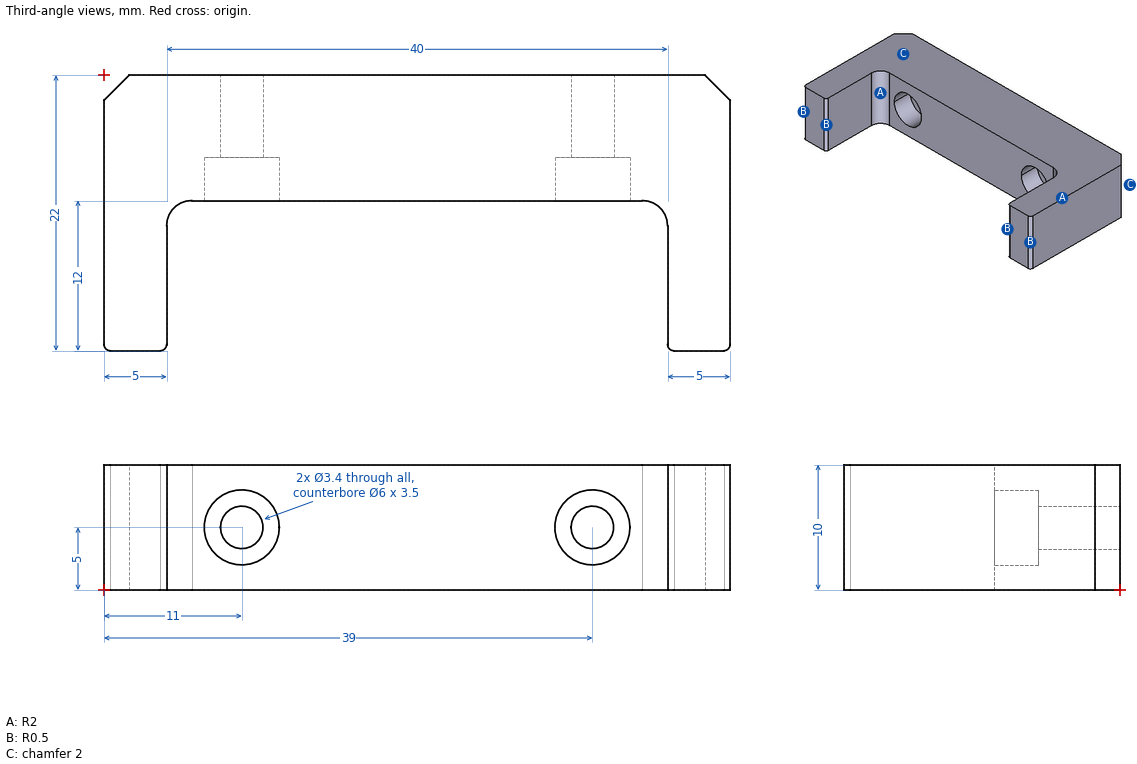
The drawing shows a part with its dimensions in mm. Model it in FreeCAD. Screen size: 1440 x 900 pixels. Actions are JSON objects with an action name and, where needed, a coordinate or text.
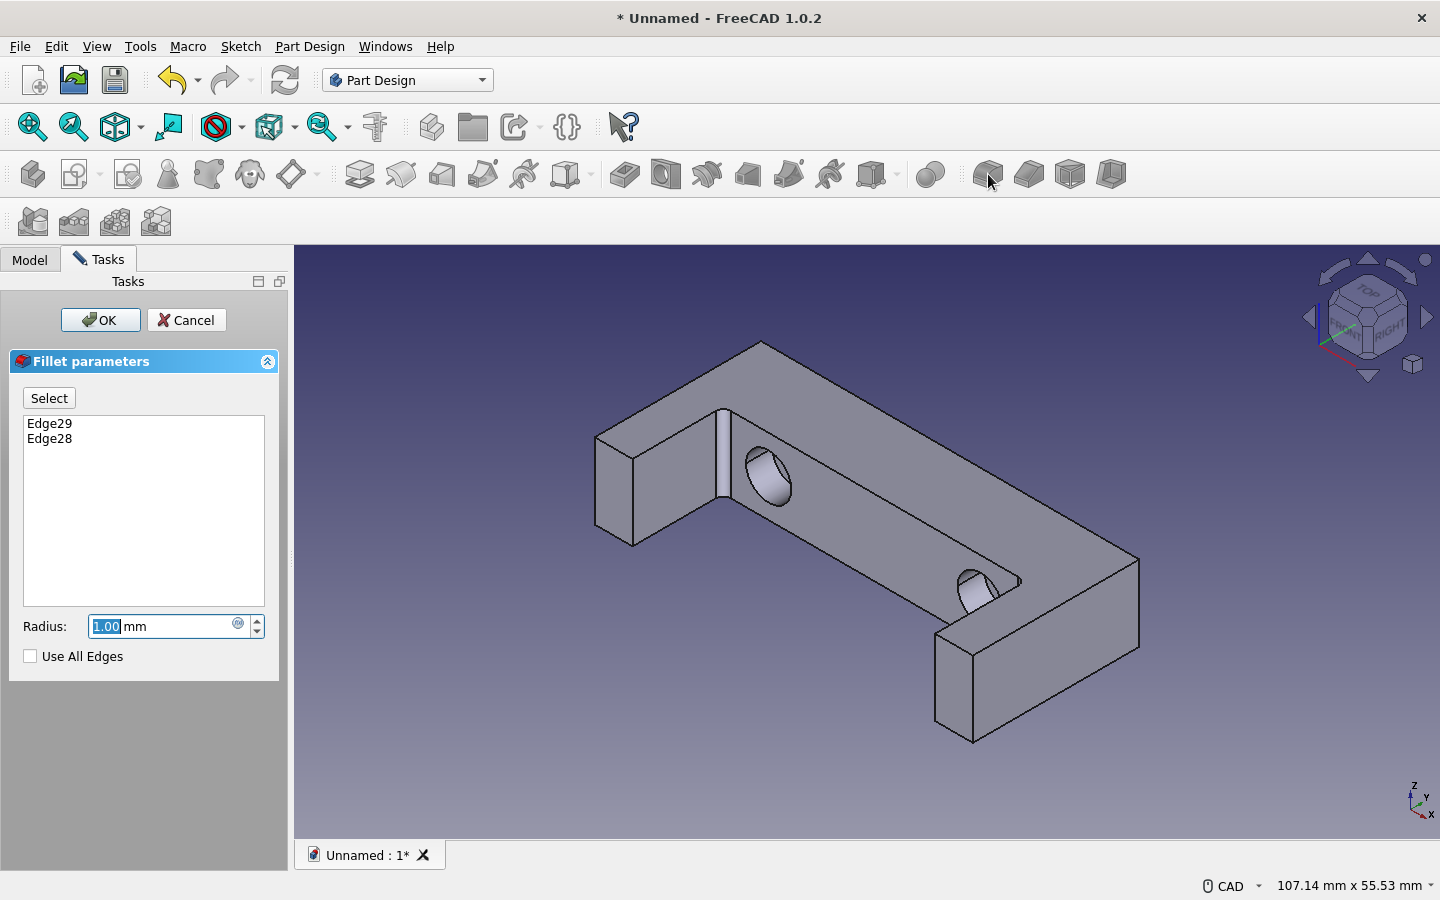
{"action": "type", "text": "2"}
{"action": "key", "text": "Tab"}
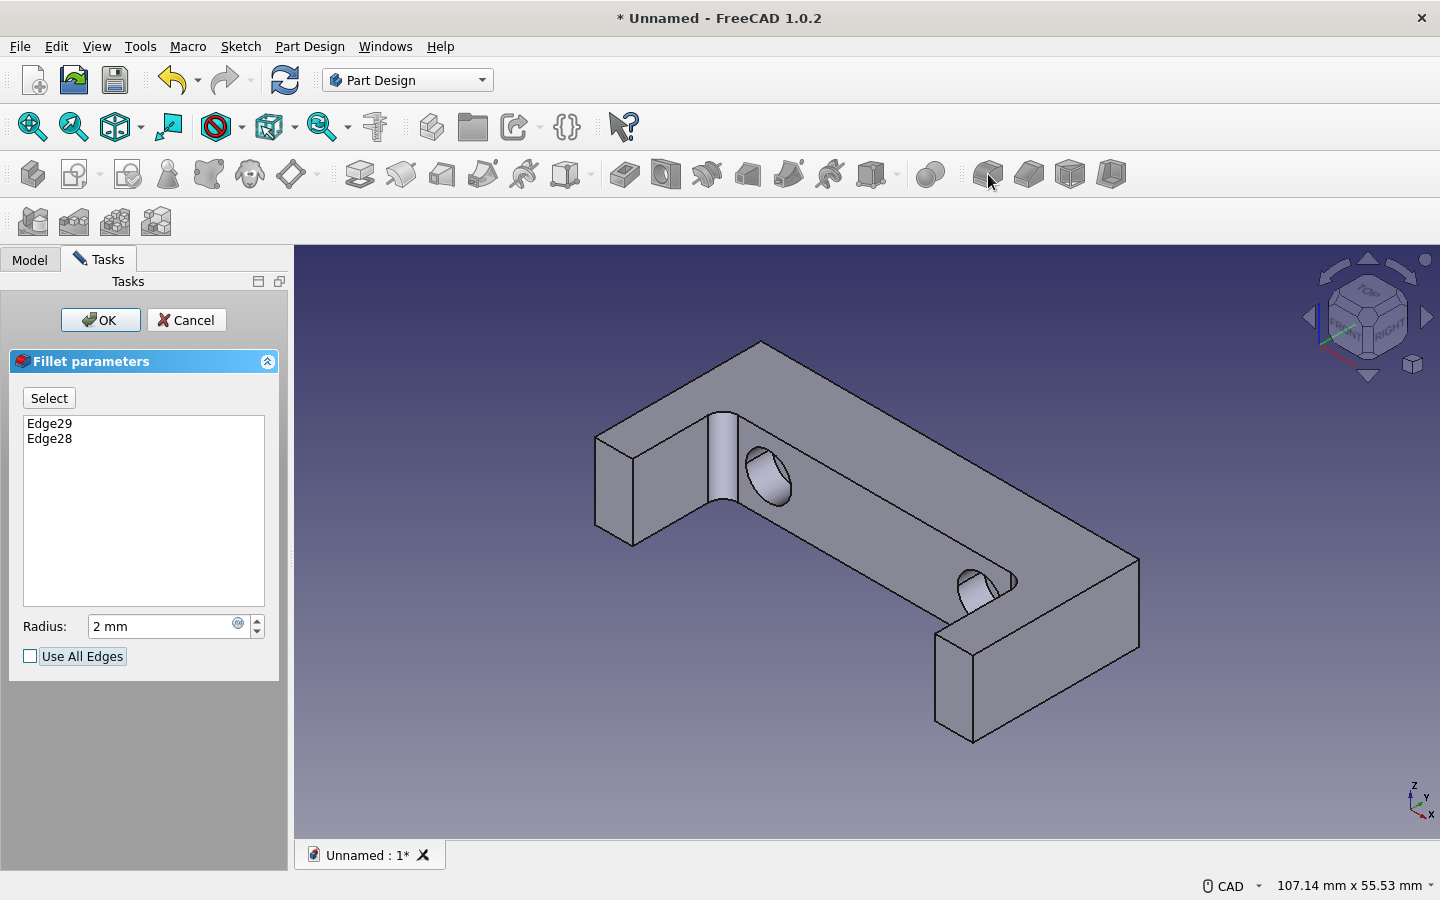
{"action": "left_click", "coordinate": [101, 320]}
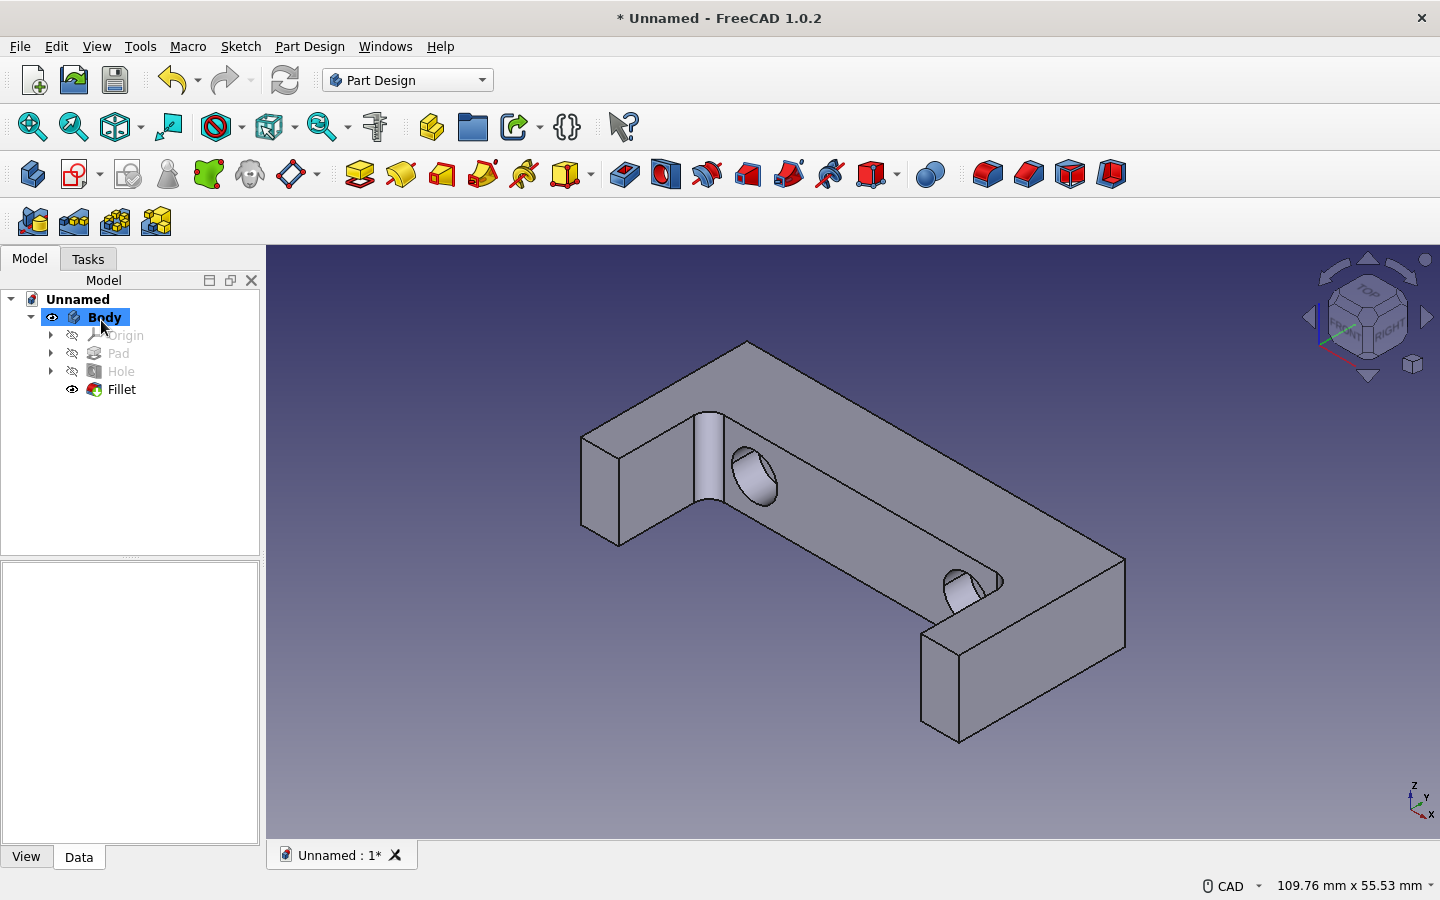
{"action": "left_click", "coordinate": [959, 698]}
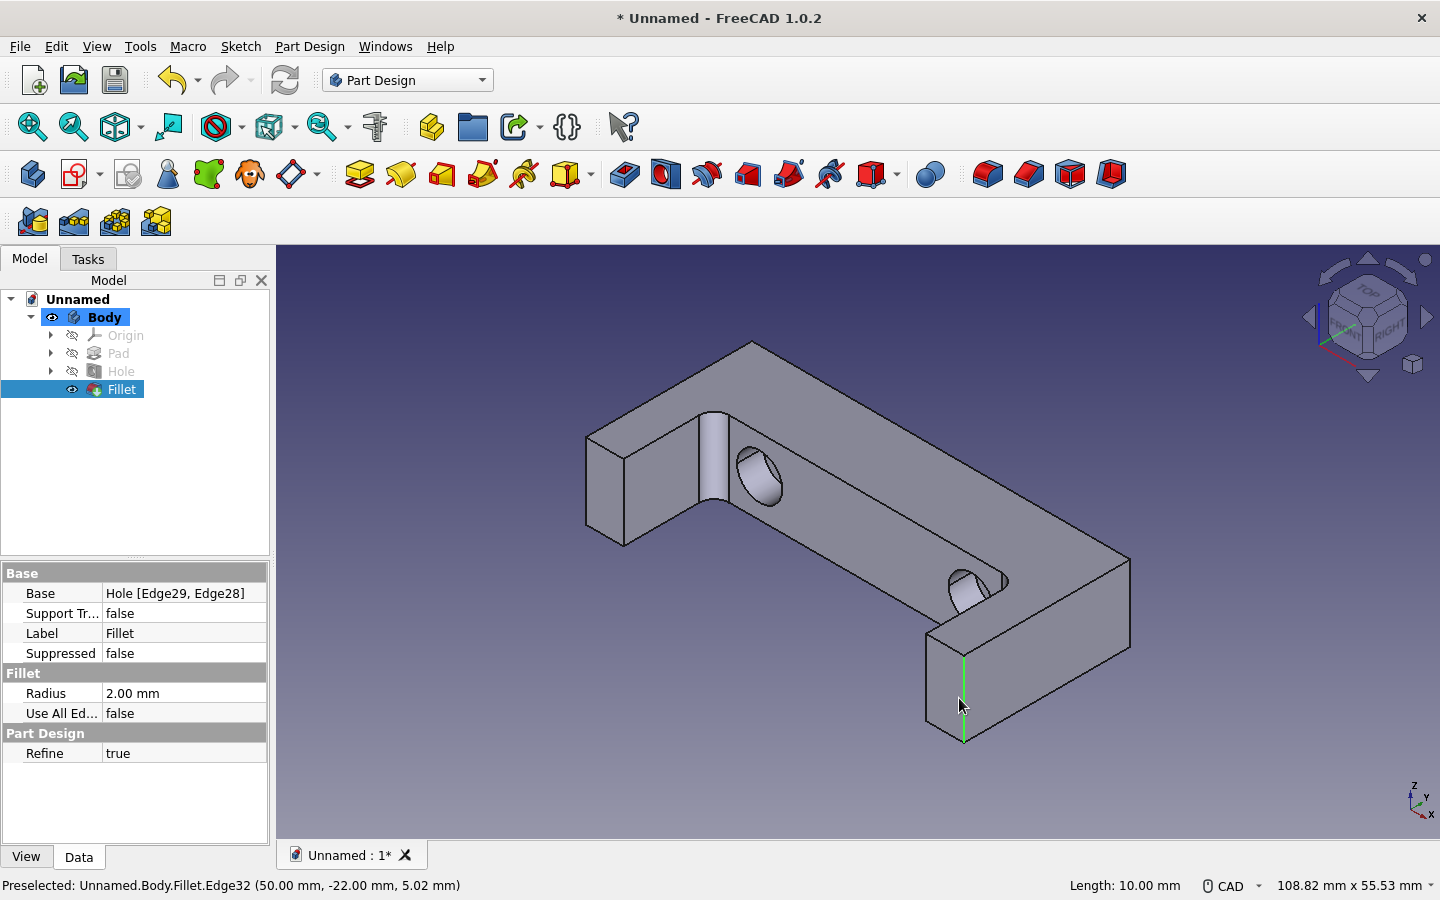
{"action": "left_click", "coordinate": [624, 502], "text": "ctrl"}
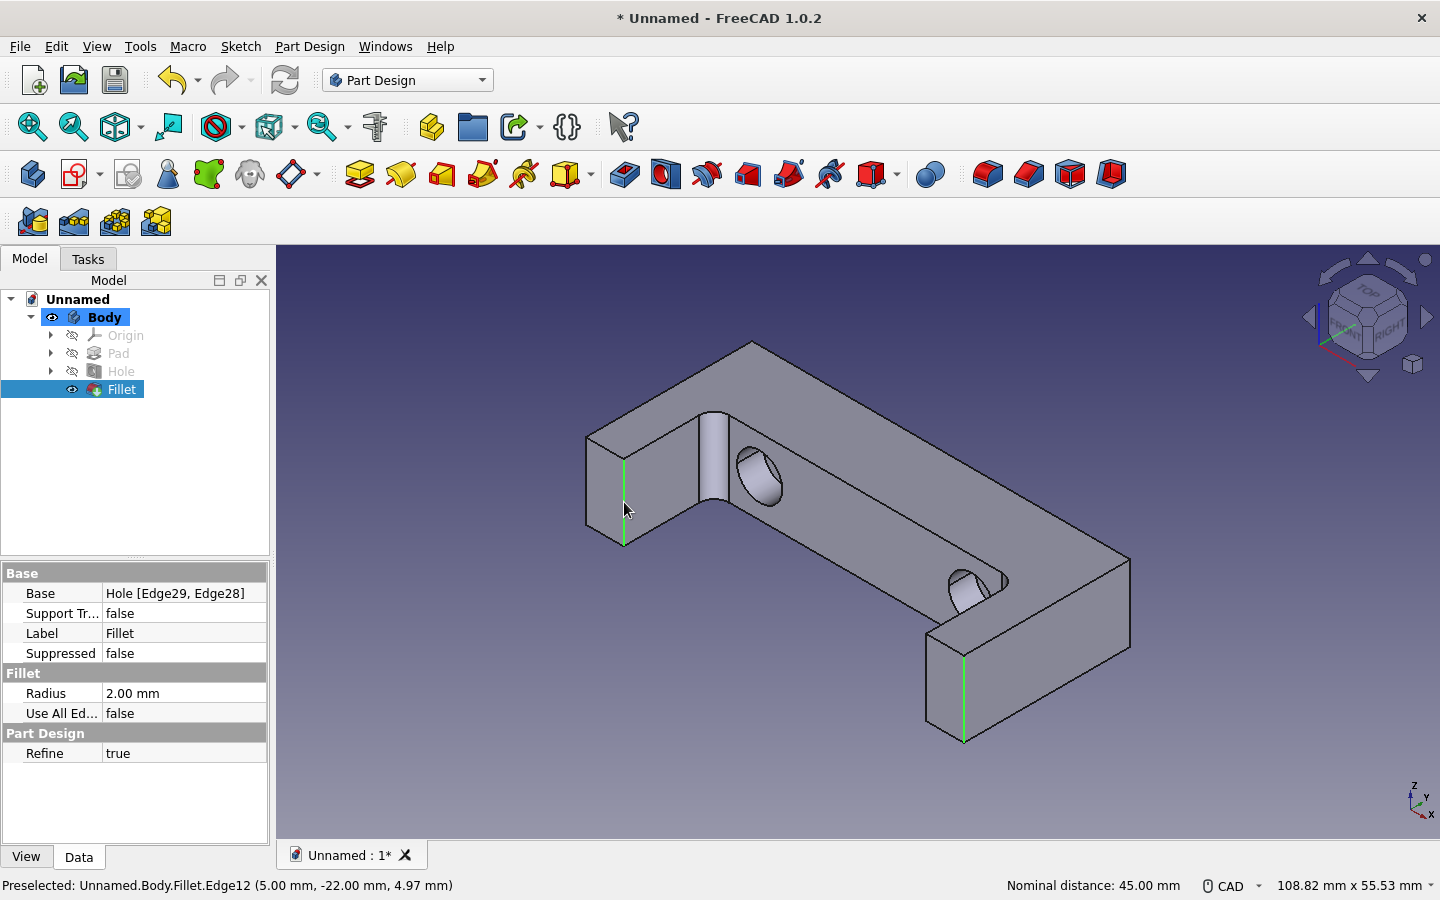
{"action": "key", "text": "2"}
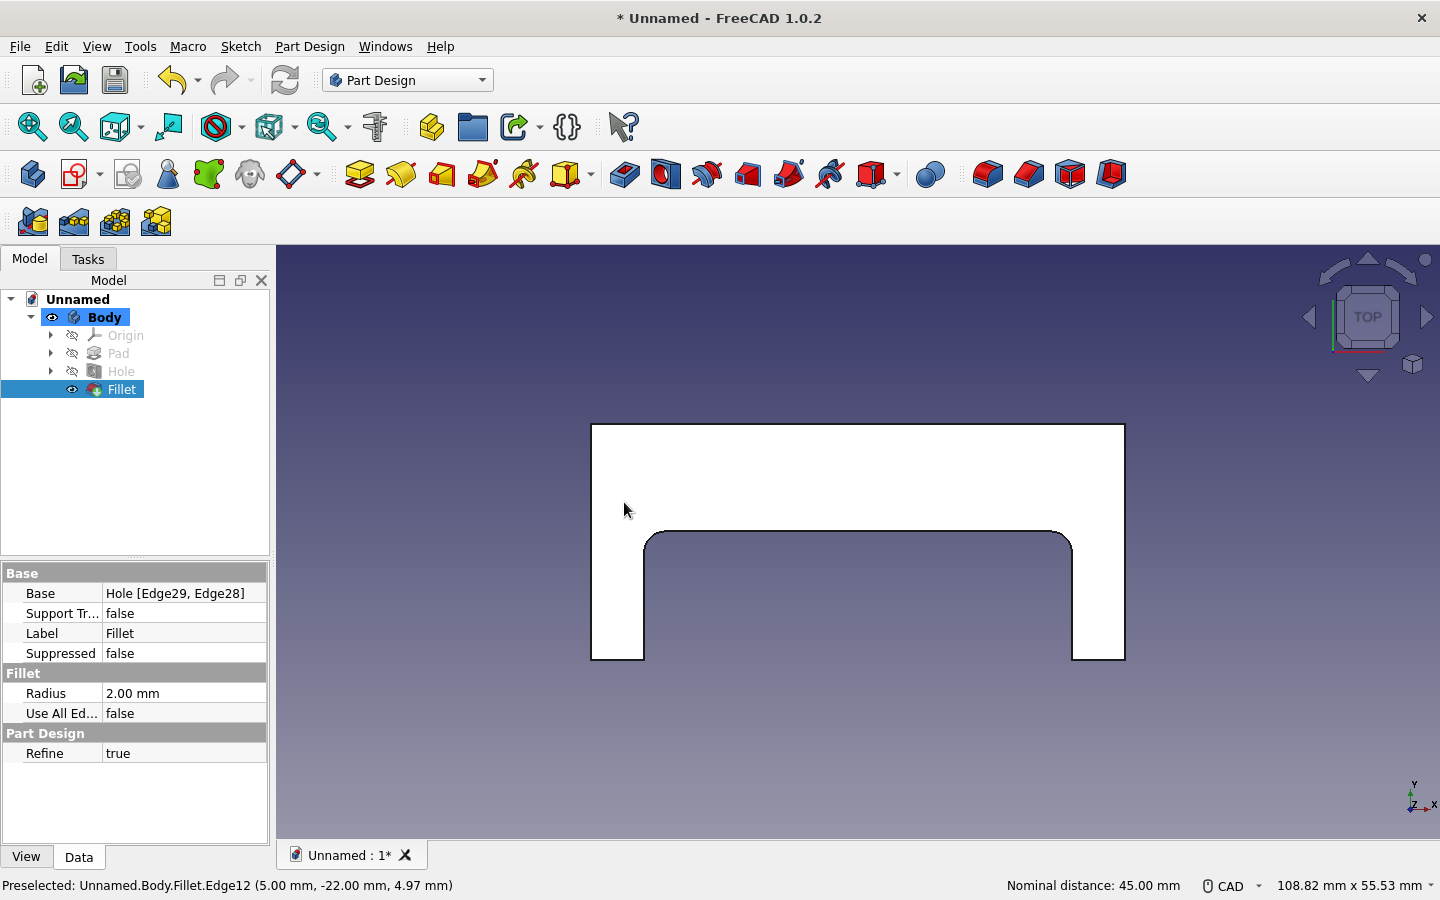
{"action": "key", "text": "0"}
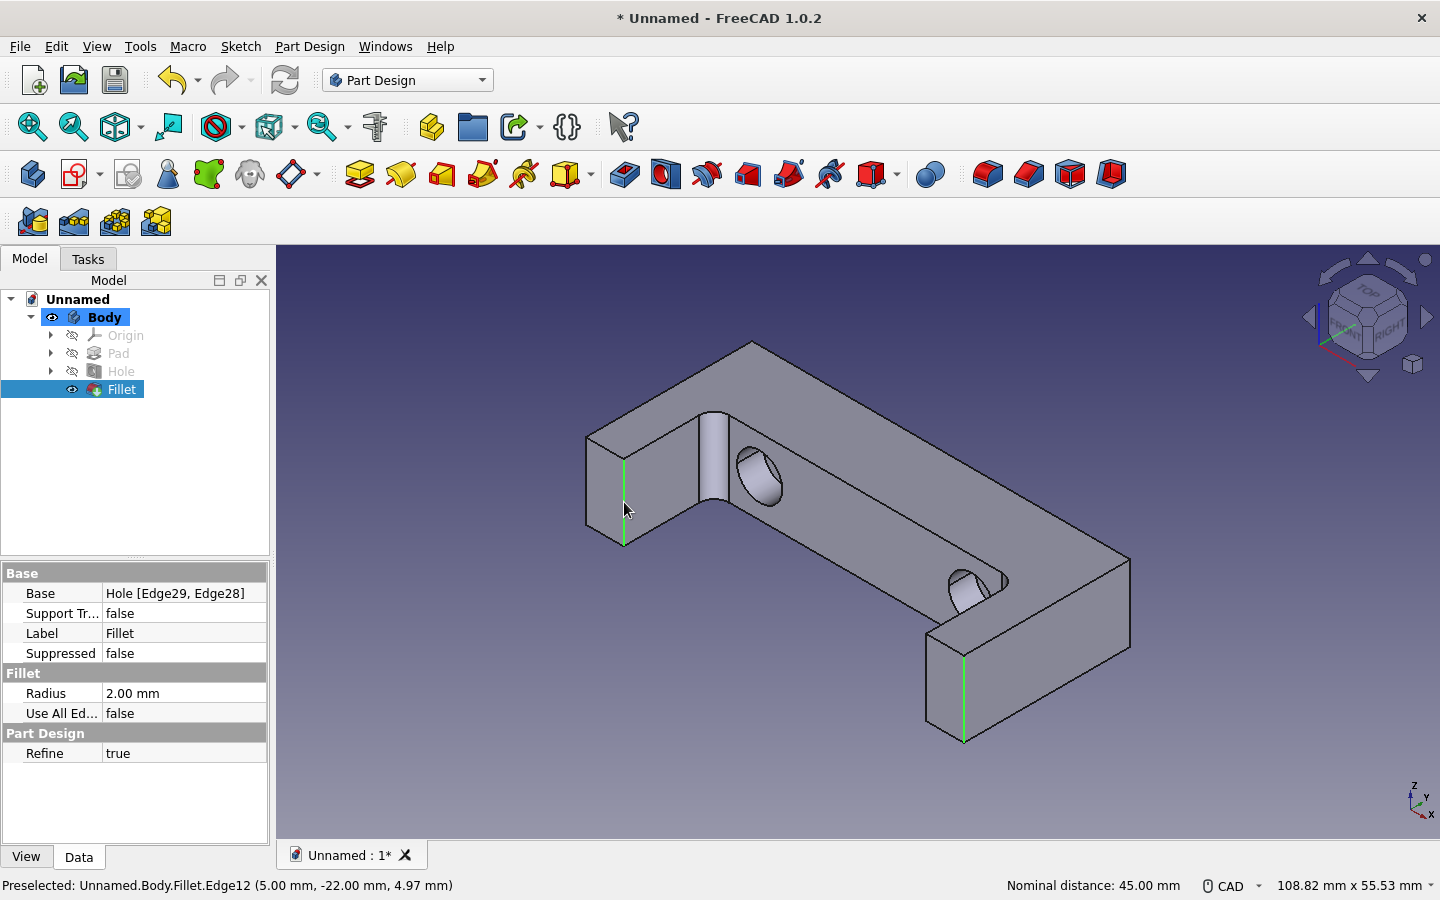
{"action": "key", "text": "1"}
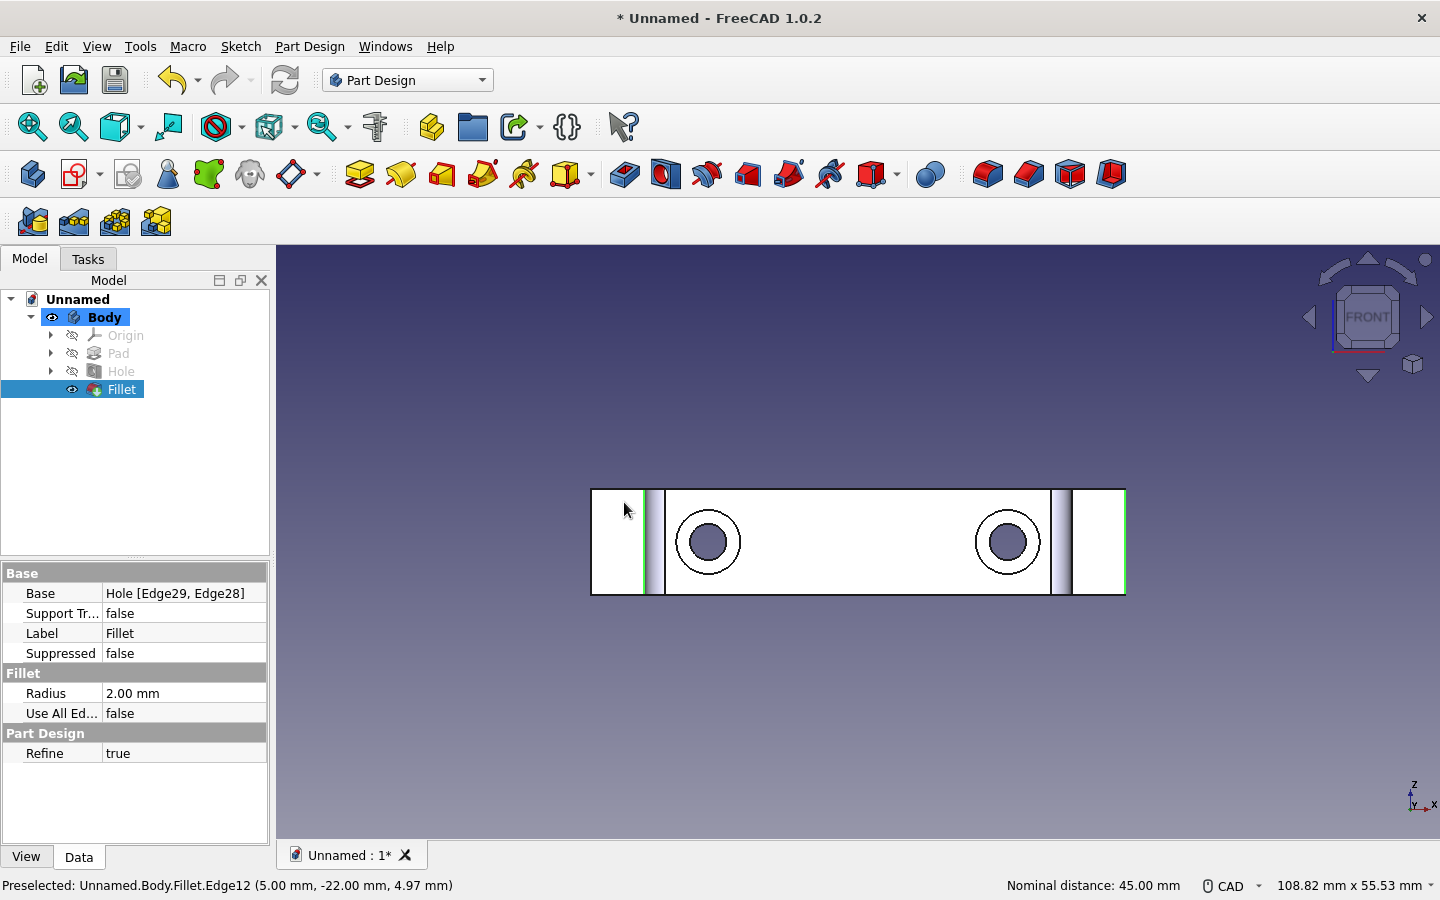
{"action": "left_click", "coordinate": [1072, 541], "text": "ctrl"}